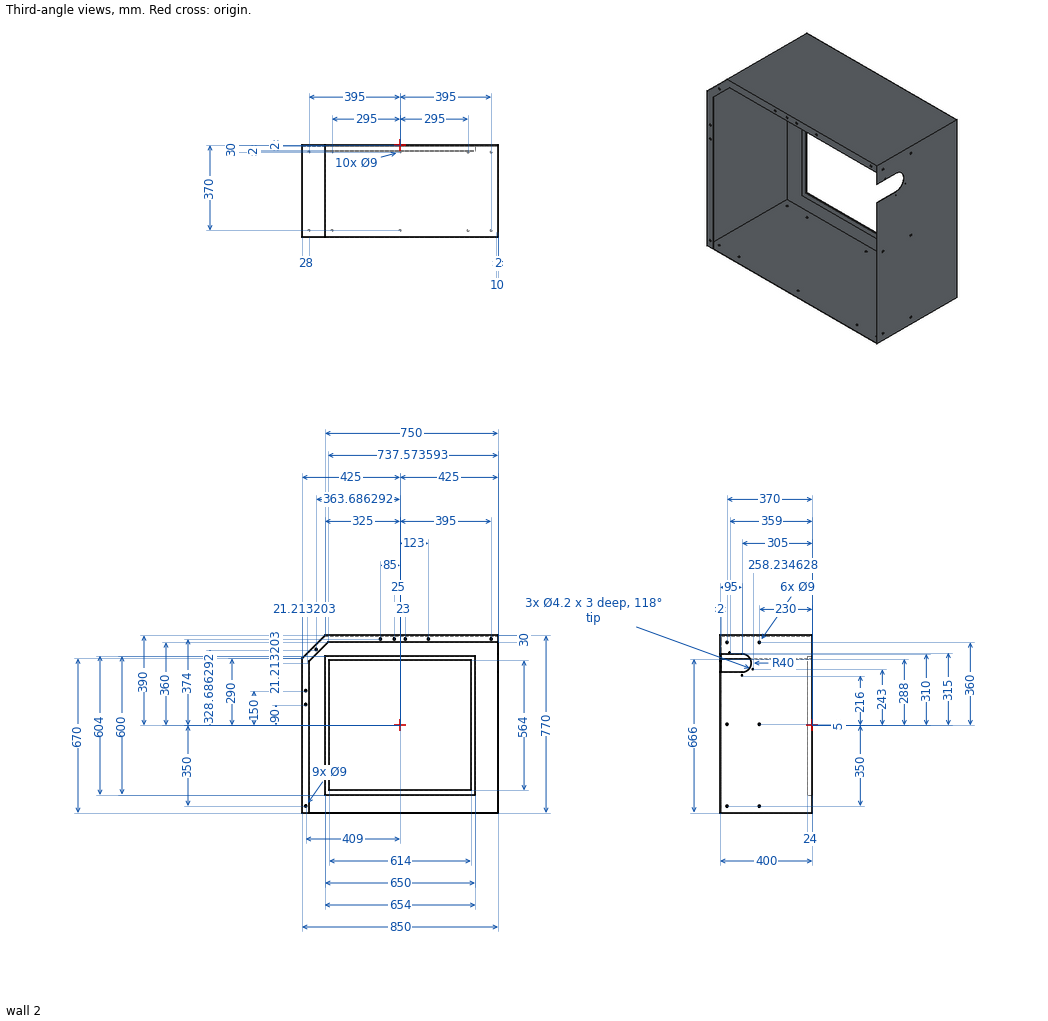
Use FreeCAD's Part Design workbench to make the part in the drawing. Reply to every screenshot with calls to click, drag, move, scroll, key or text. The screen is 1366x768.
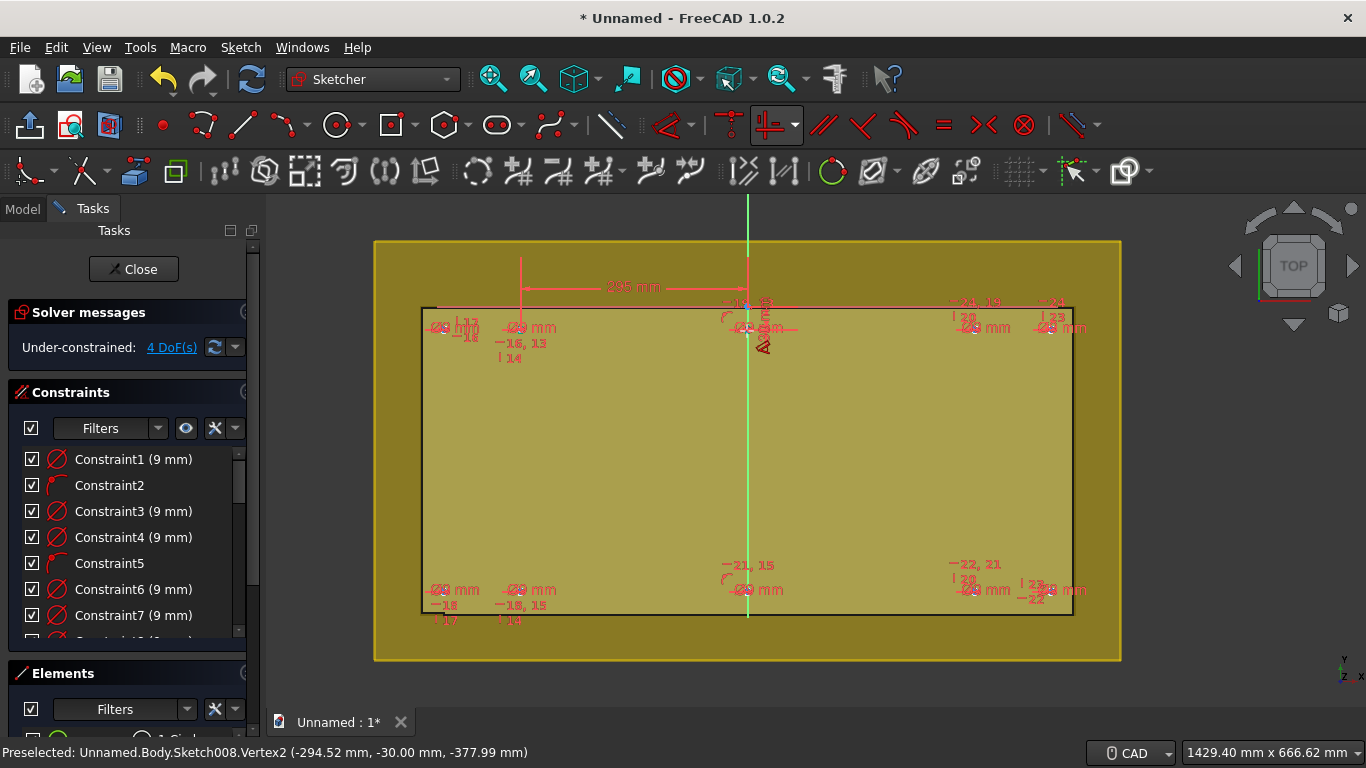
click(748, 592)
click(782, 449)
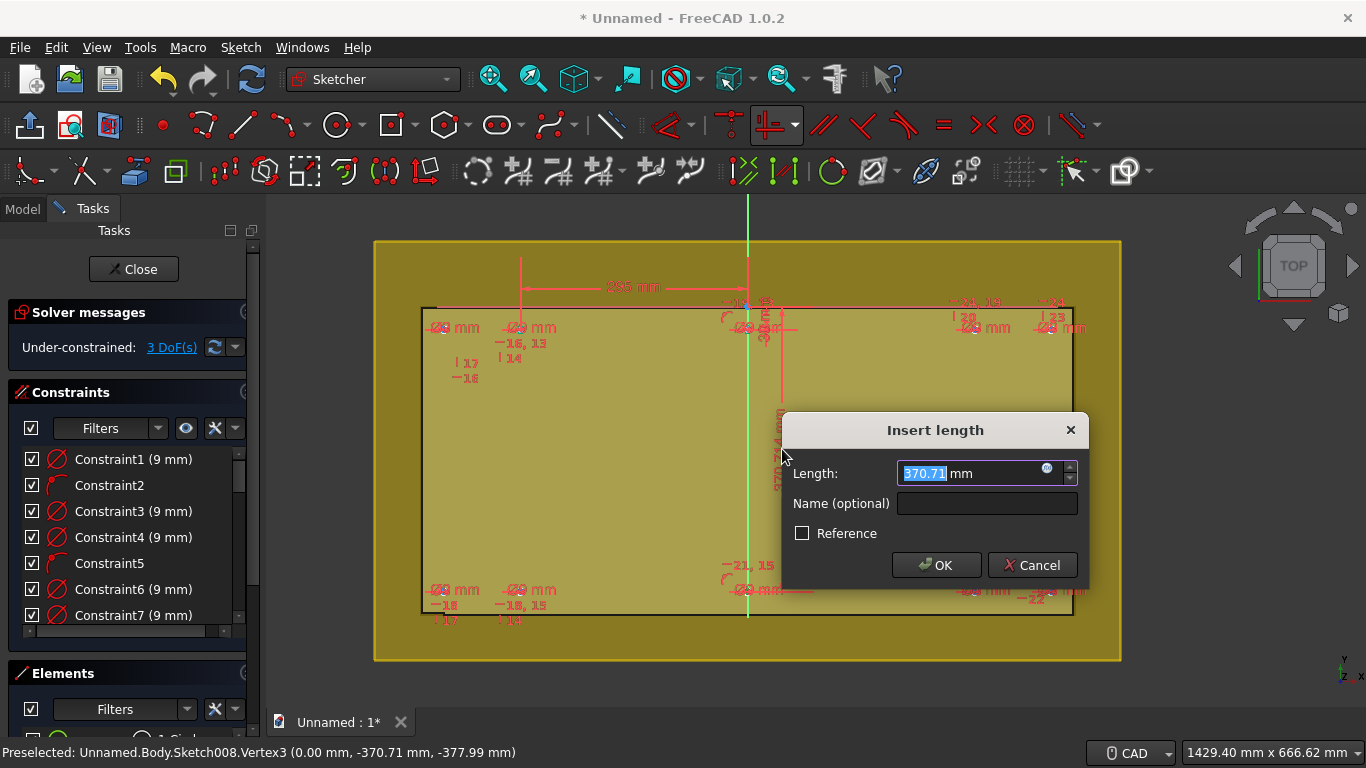
text(370)
key(Return)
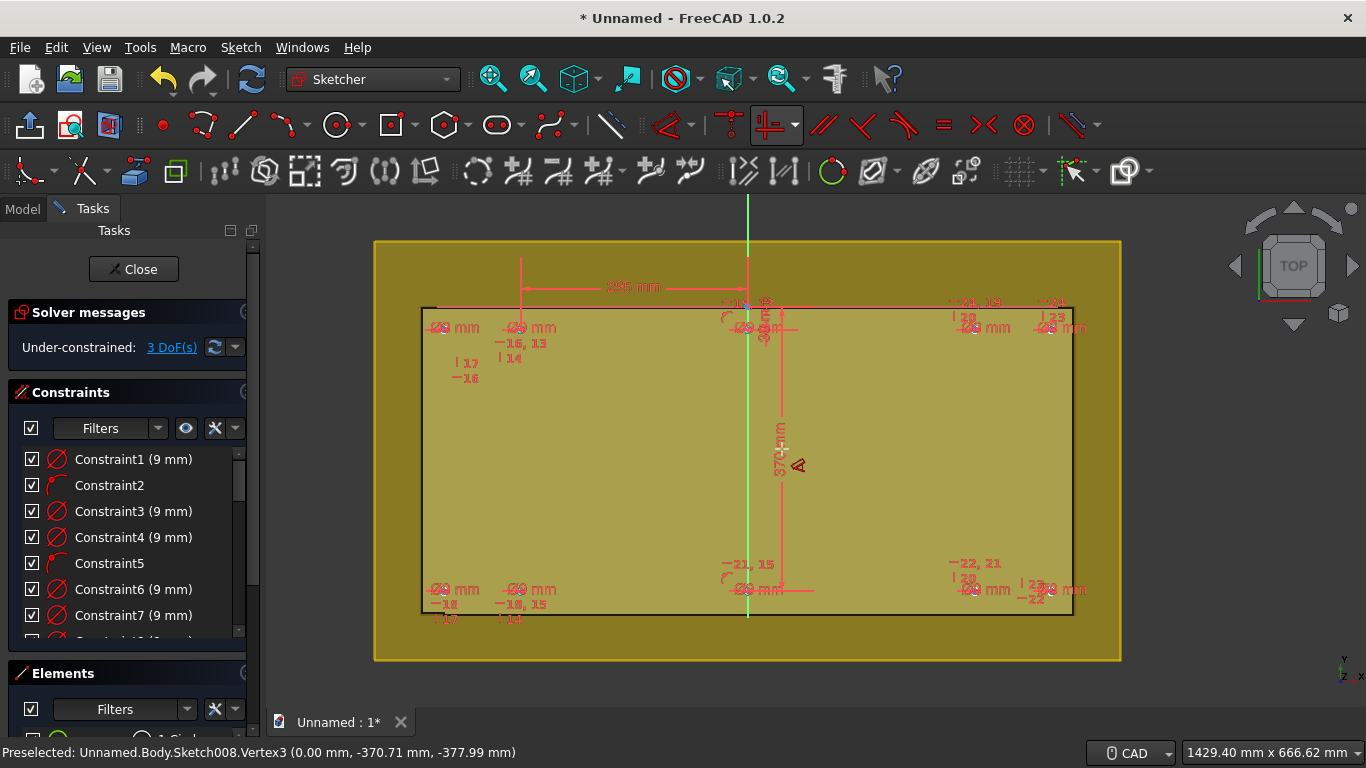
click(444, 330)
click(526, 273)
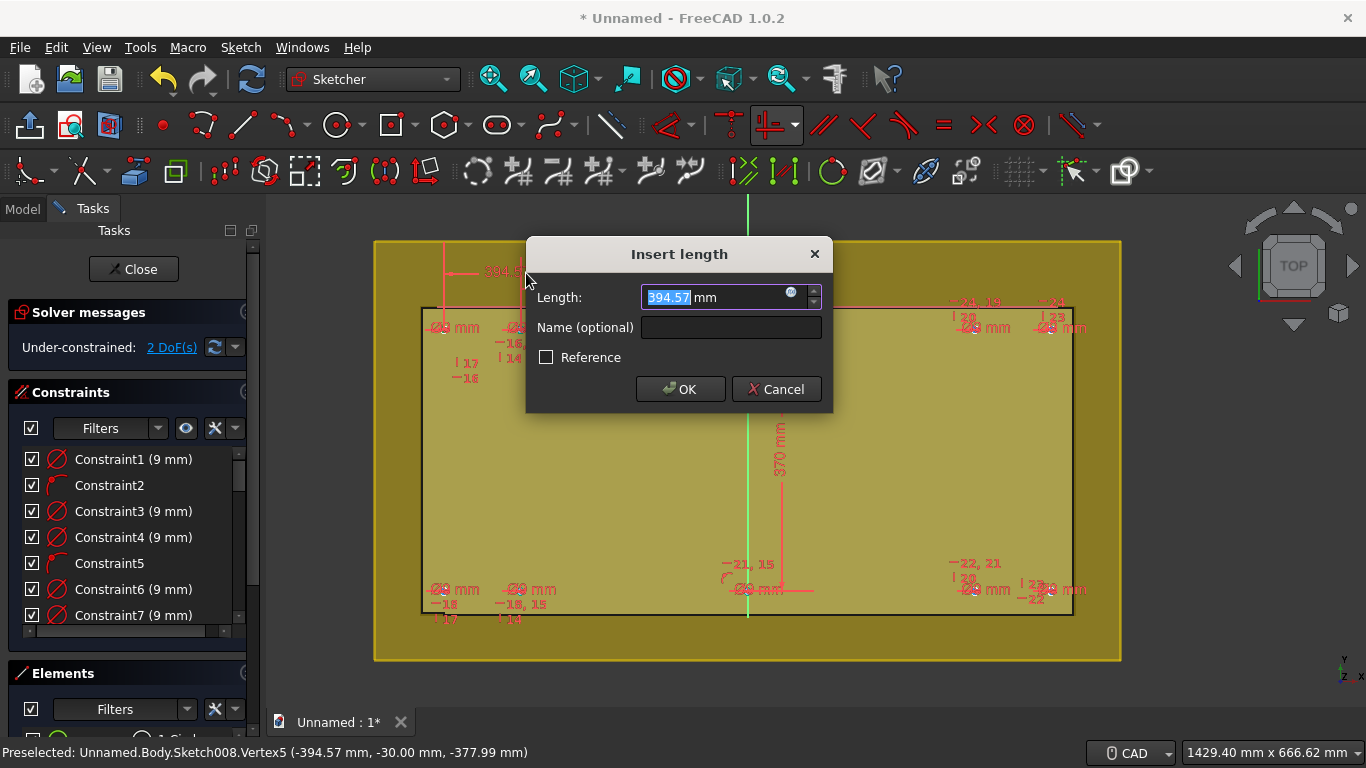
text(395)
key(Return)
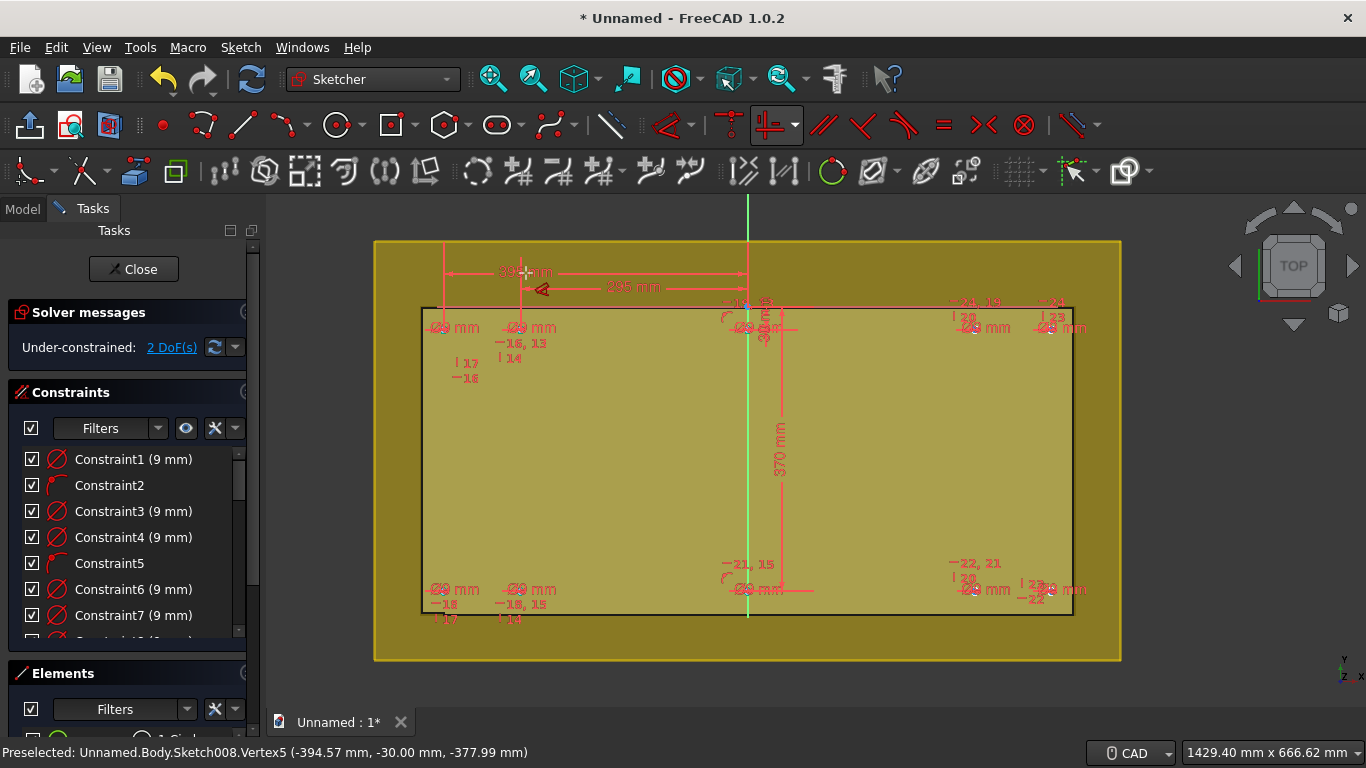
click(975, 330)
click(861, 273)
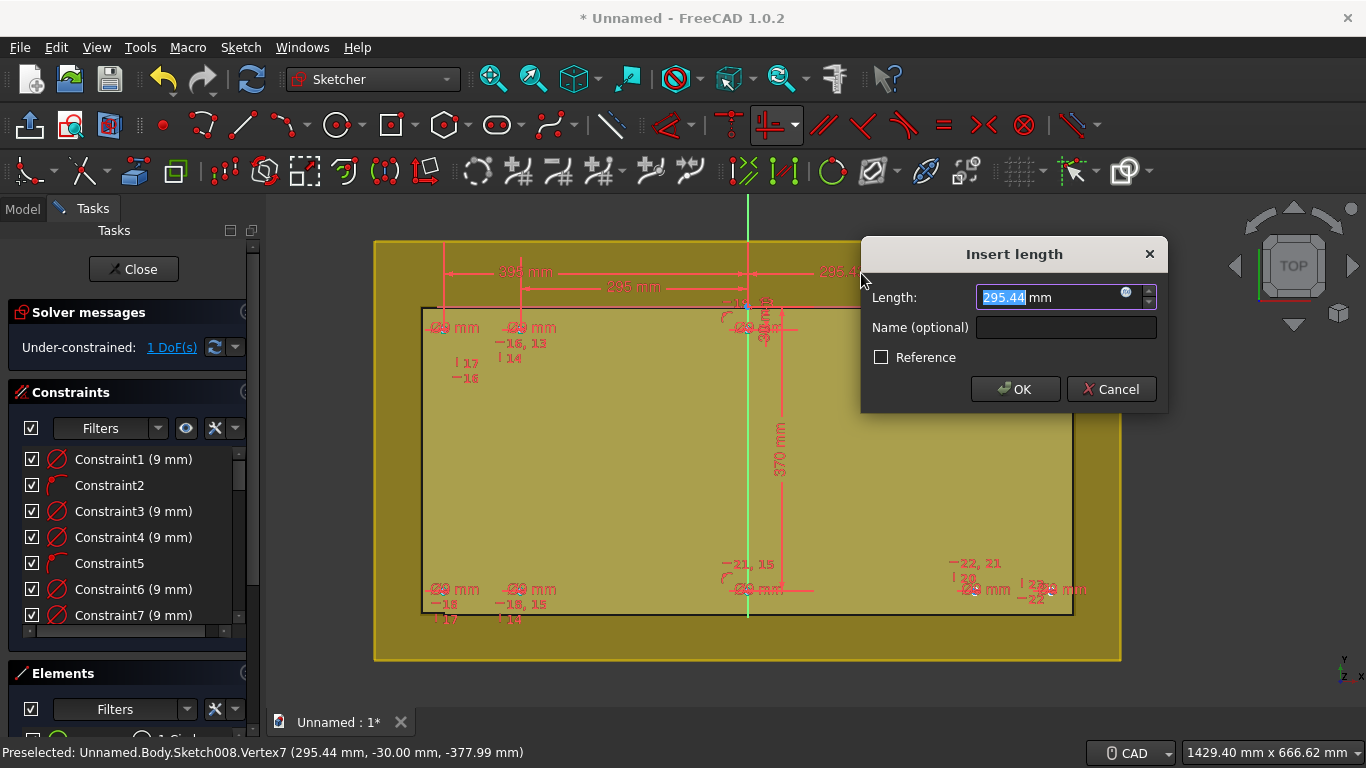
text(295)
key(Return)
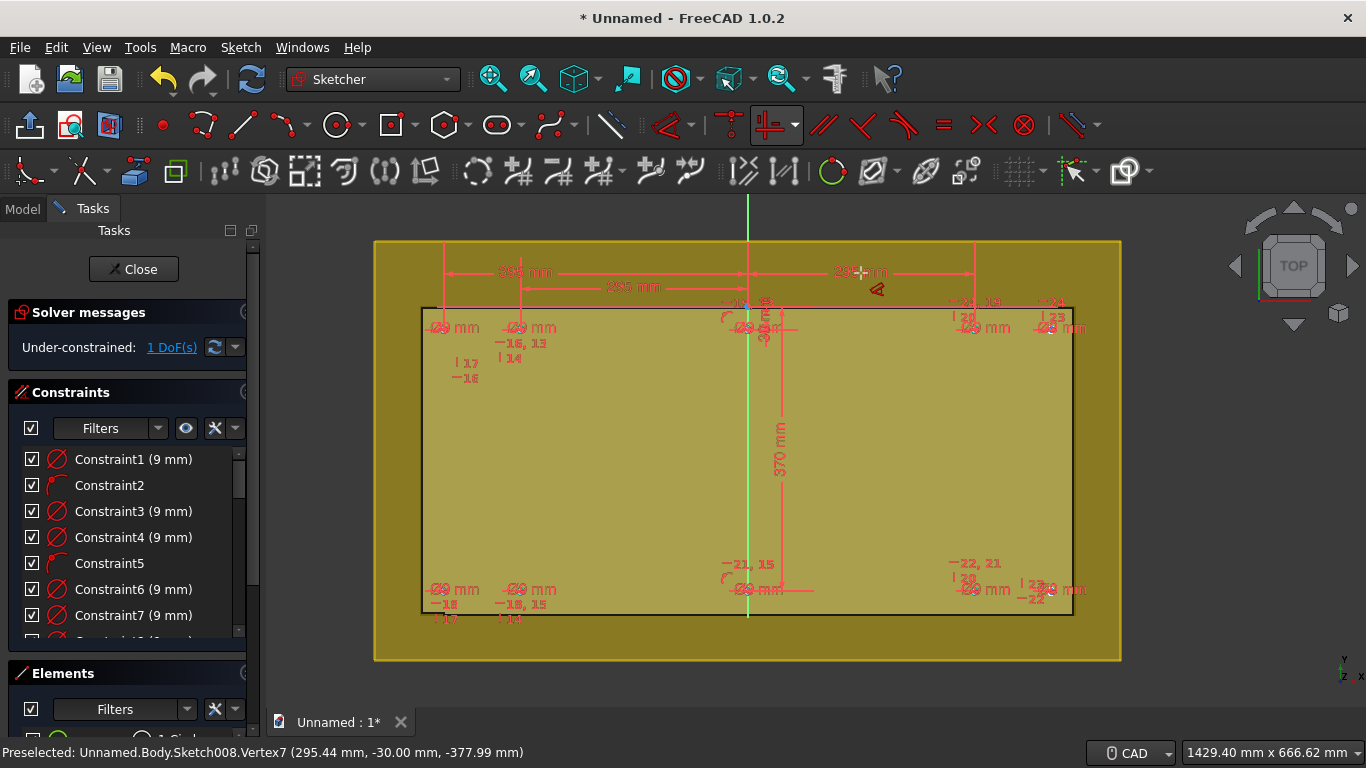
click(1051, 591)
click(969, 273)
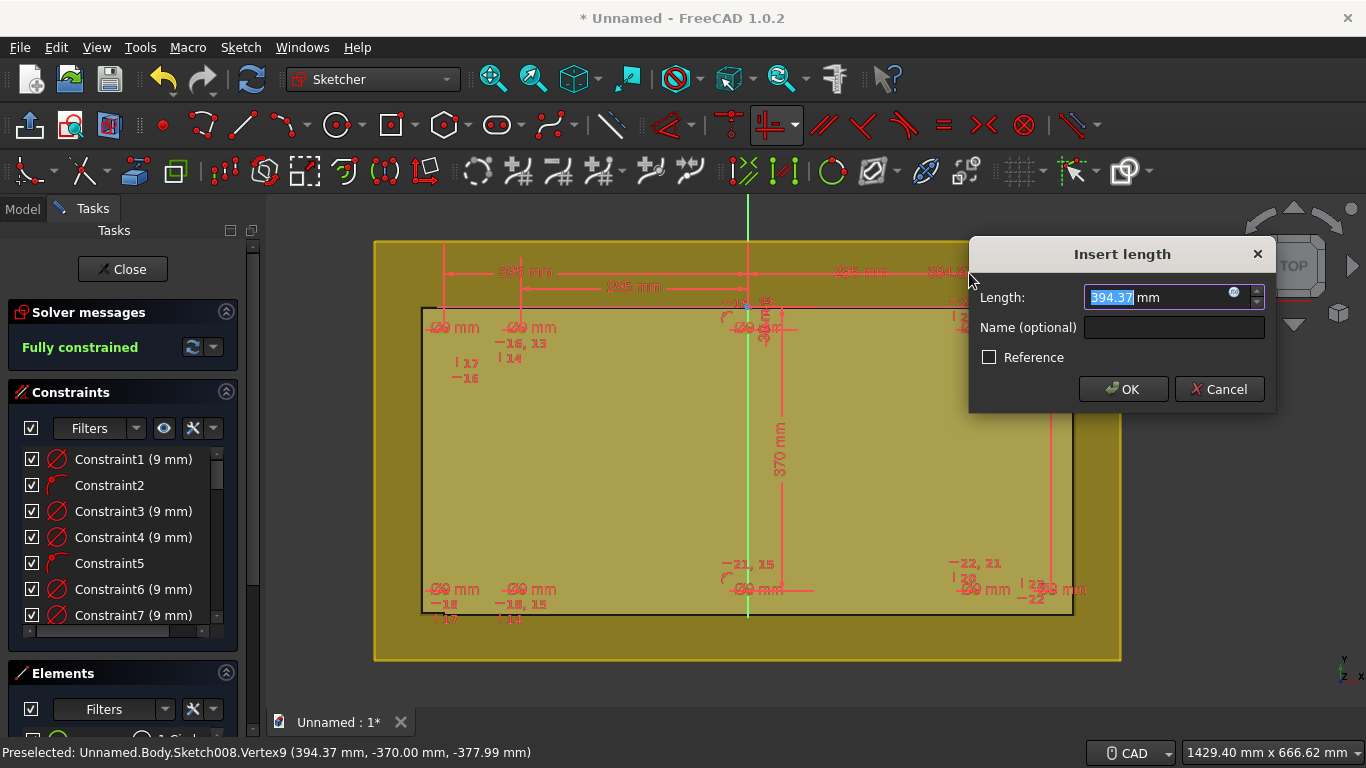
text(395)
key(Return)
key(Escape)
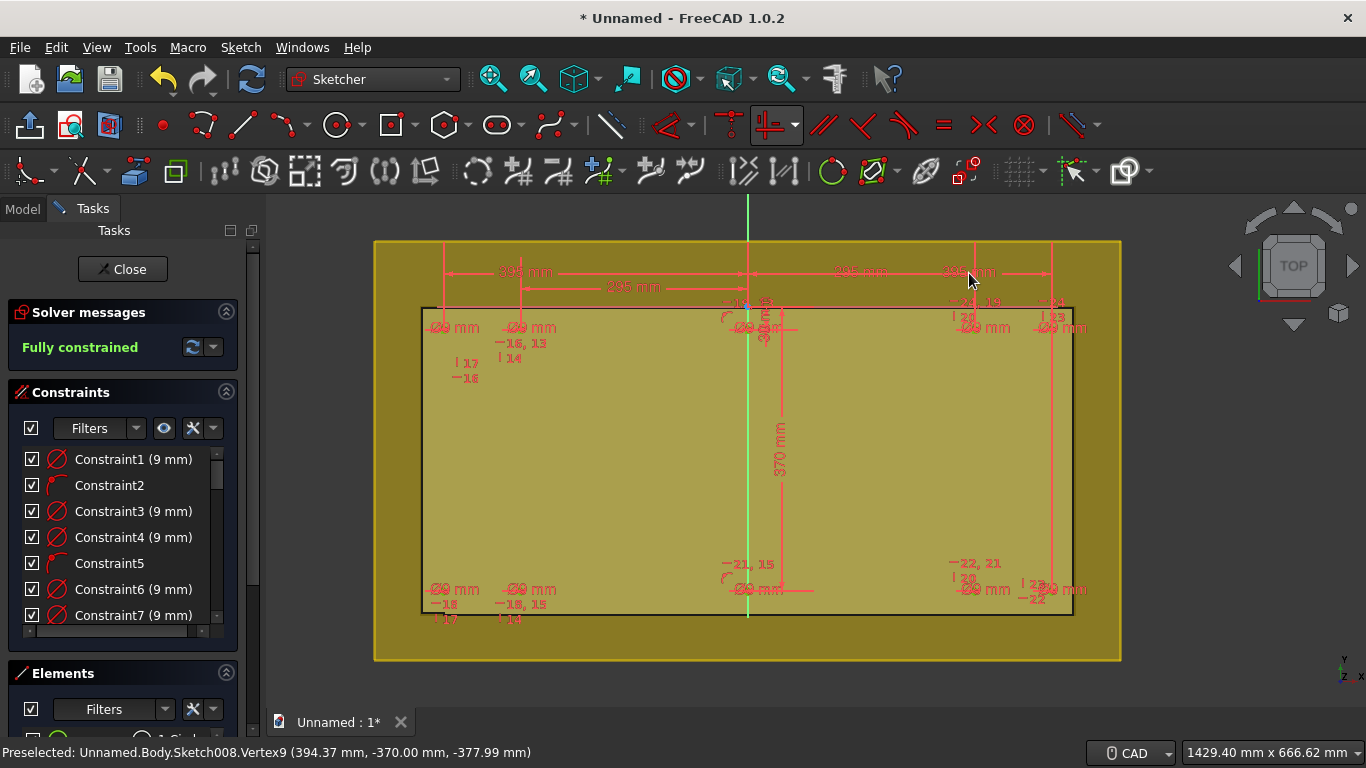
click(123, 269)